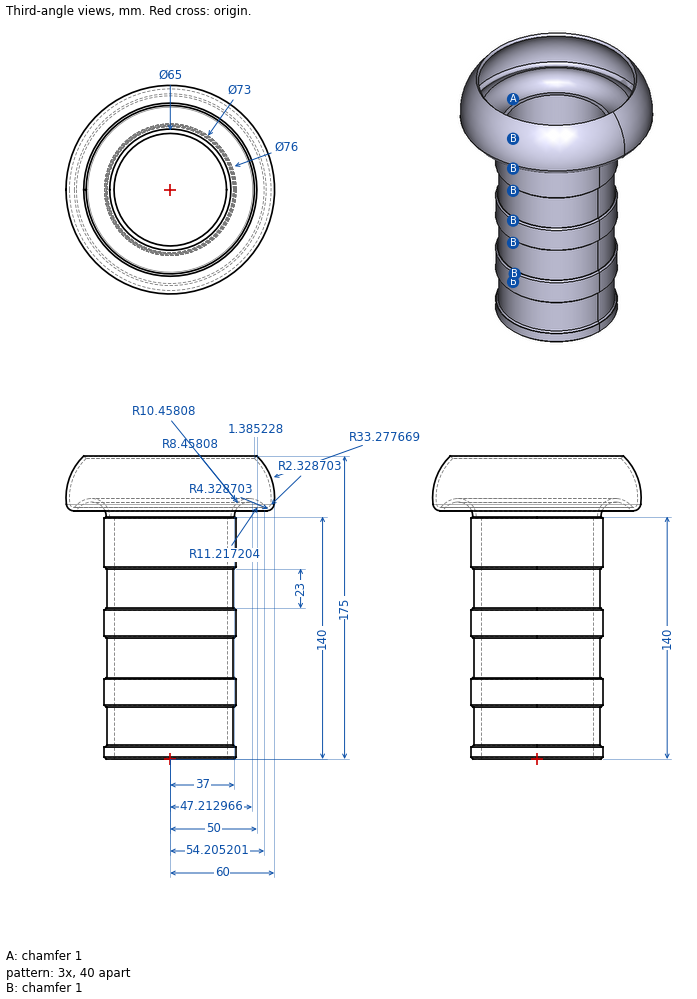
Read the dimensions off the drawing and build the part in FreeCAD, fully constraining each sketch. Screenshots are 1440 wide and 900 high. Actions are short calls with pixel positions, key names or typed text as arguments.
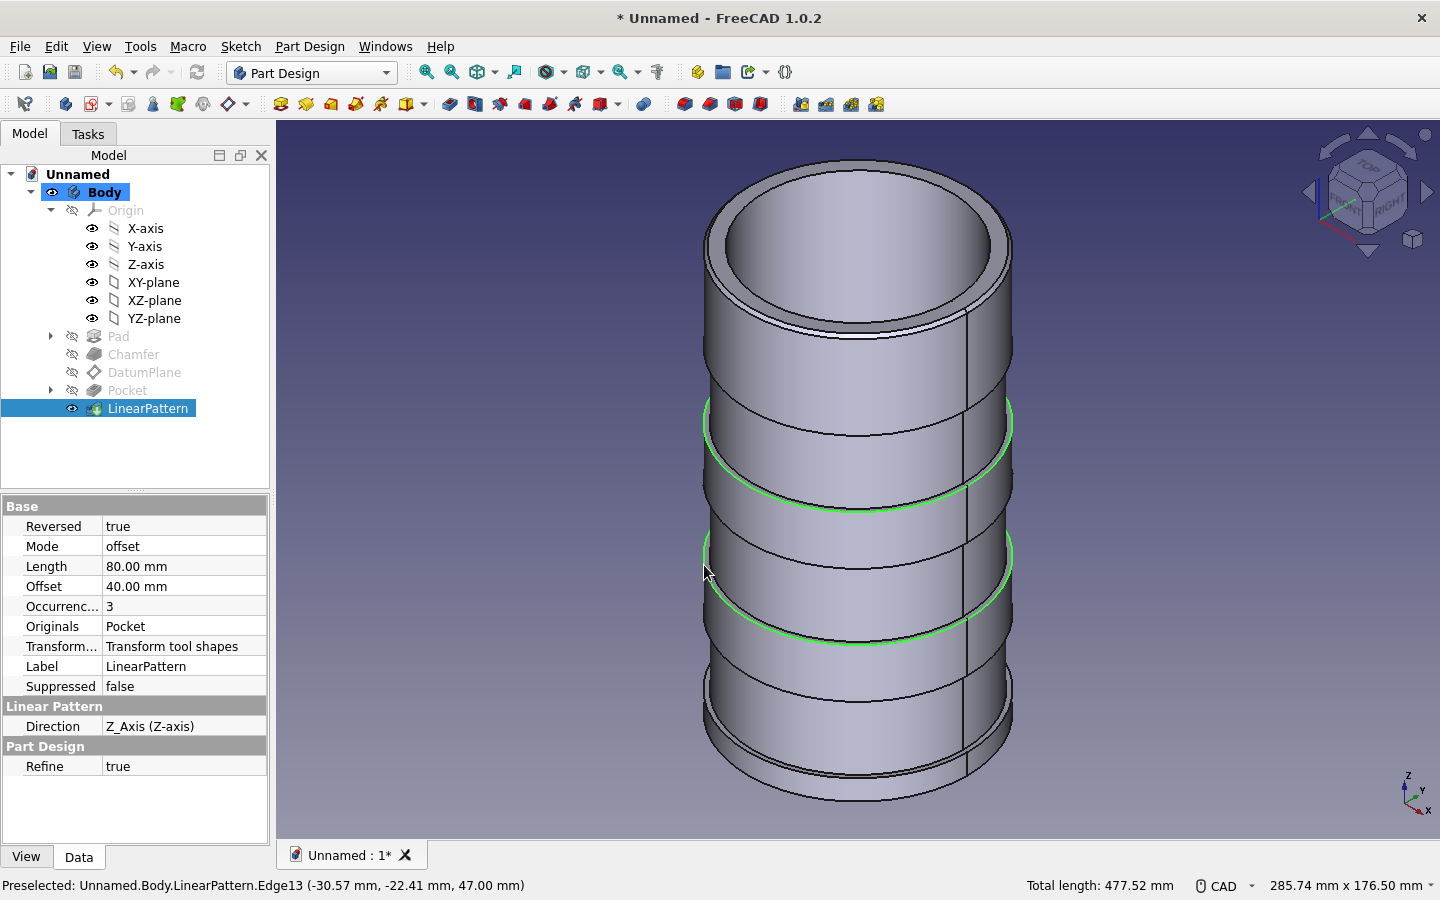
key(v)
key(f)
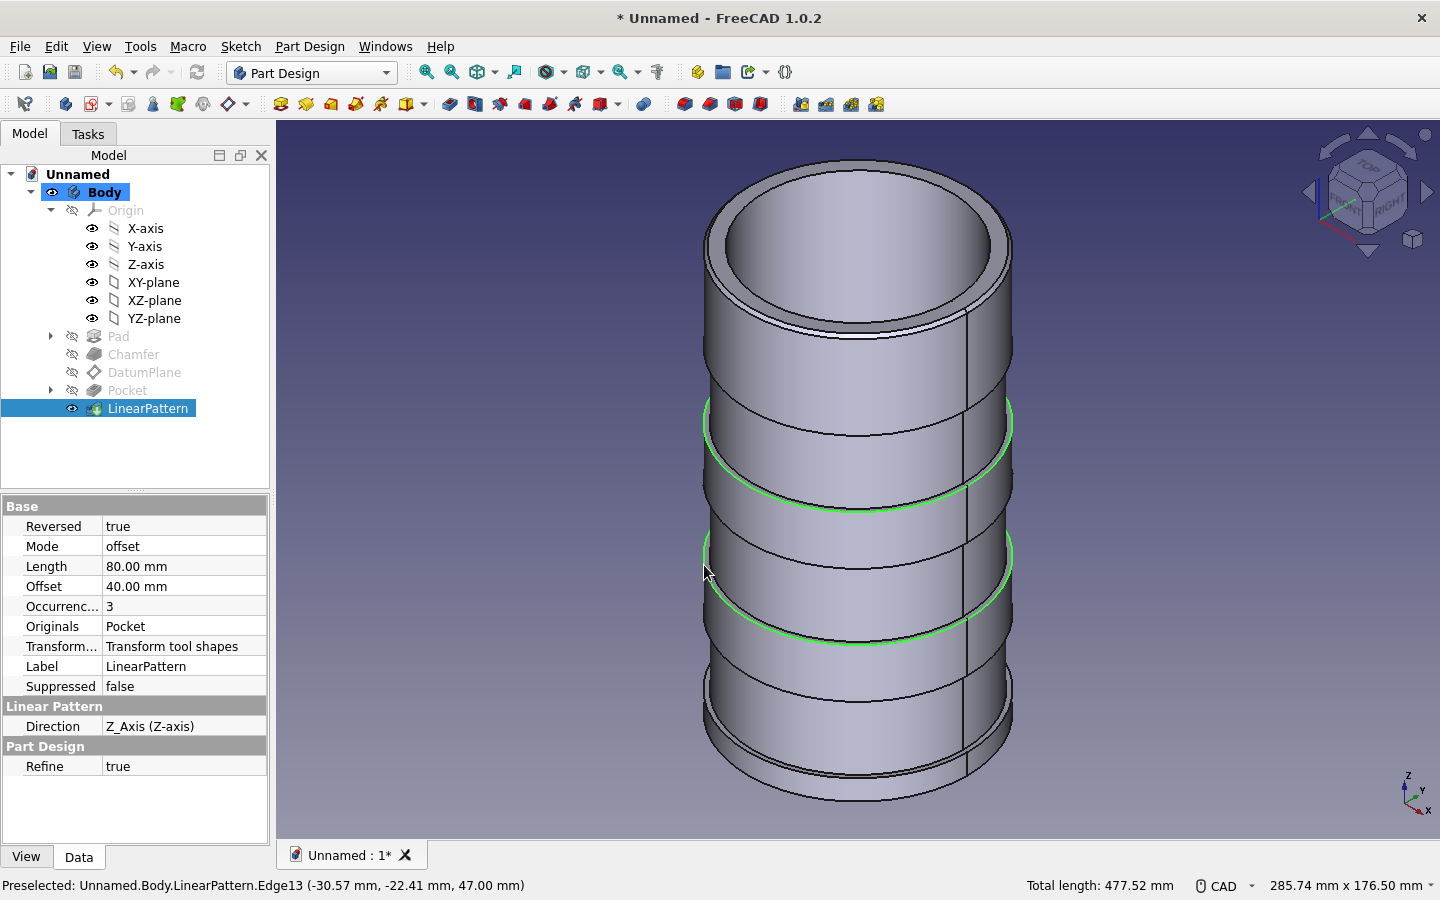
click(720, 386, ctrl)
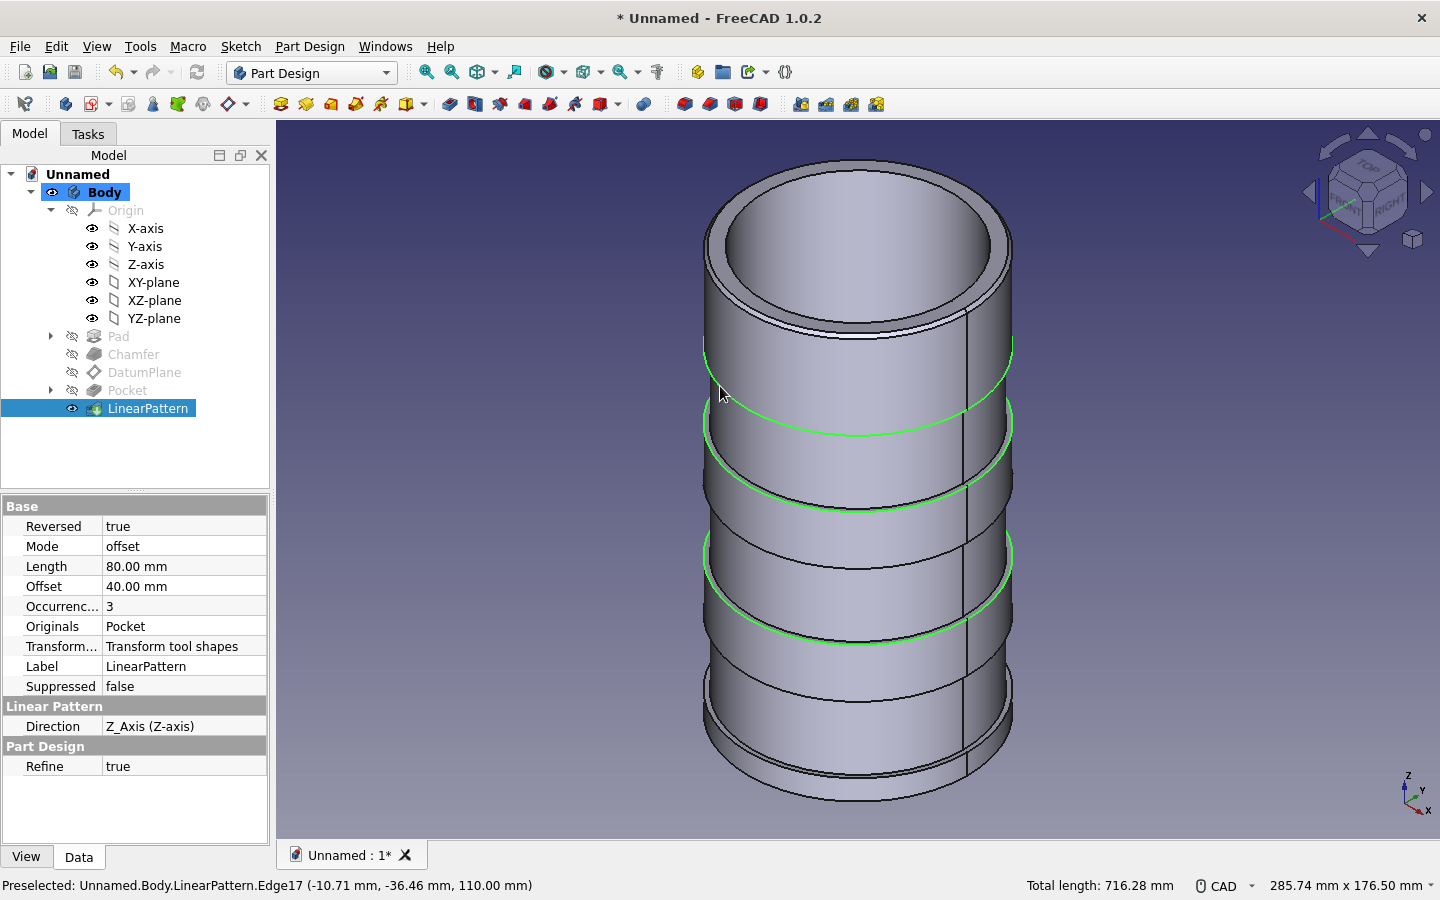
click(720, 752, ctrl)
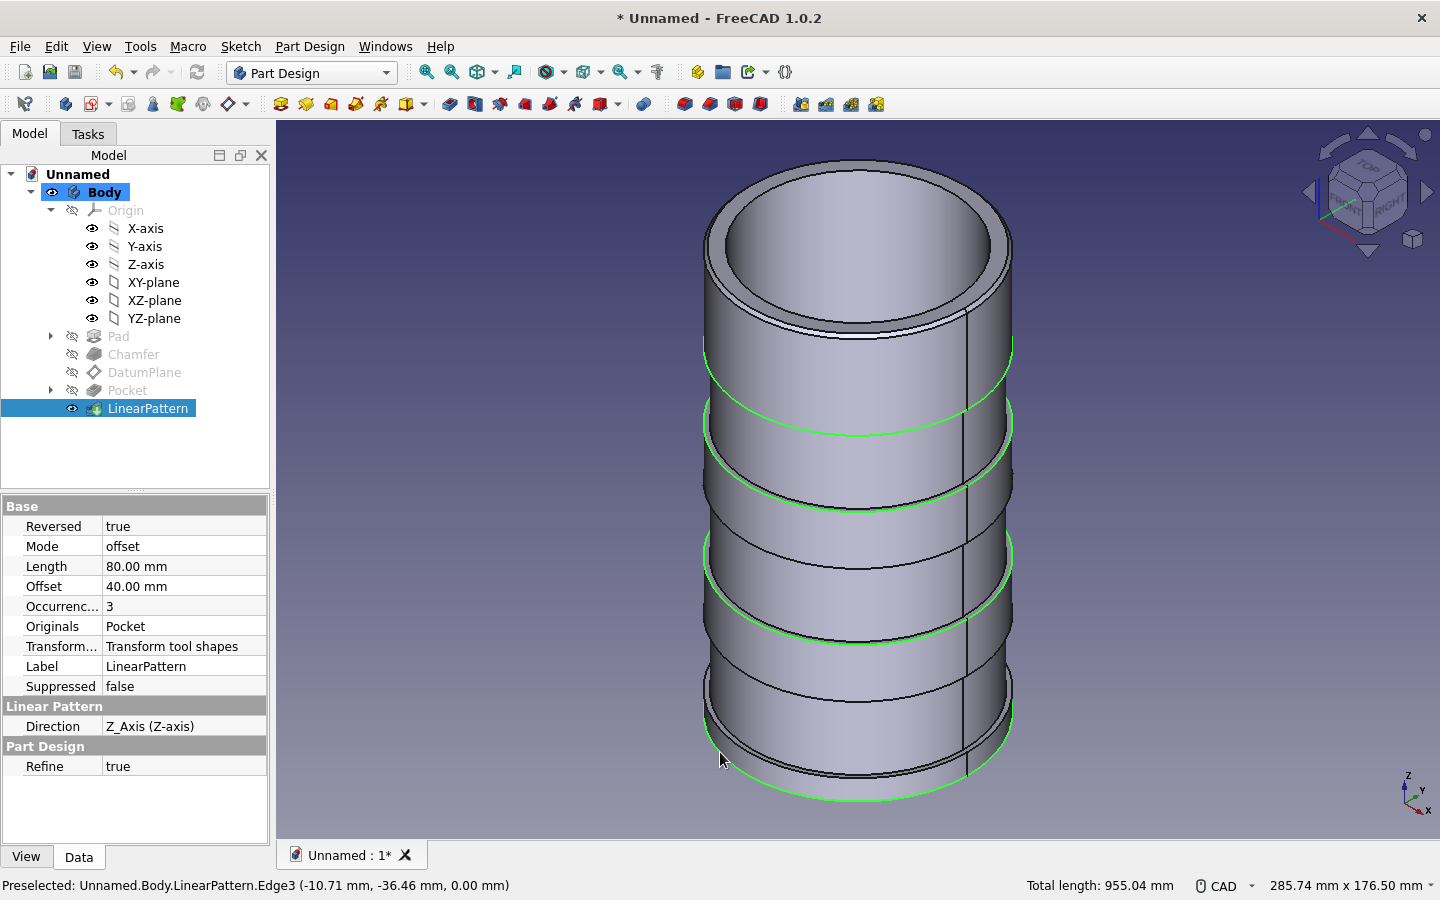
click(720, 519, ctrl)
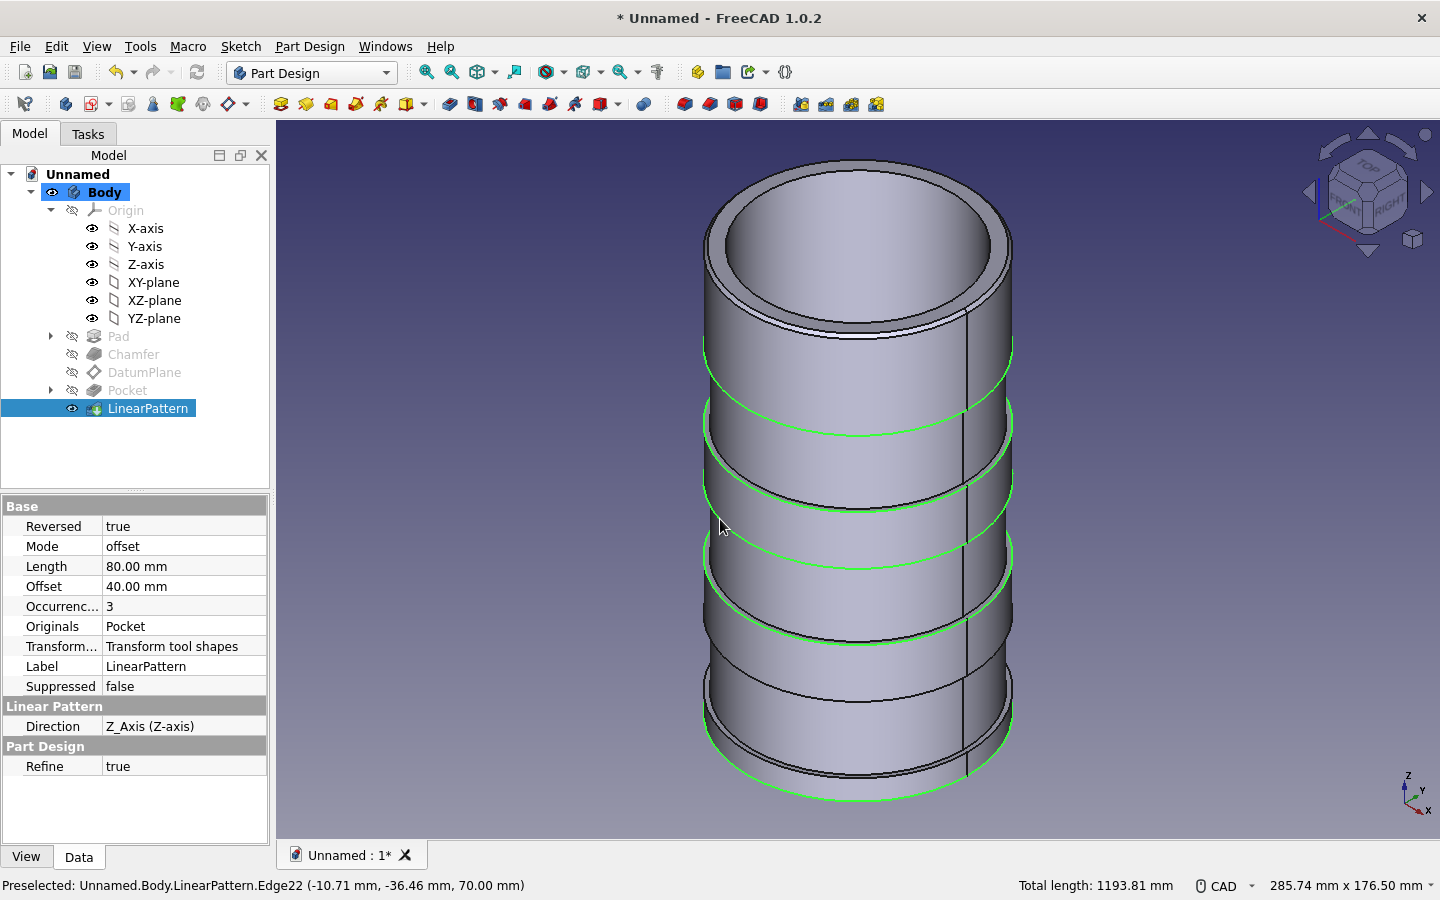
click(720, 652, ctrl)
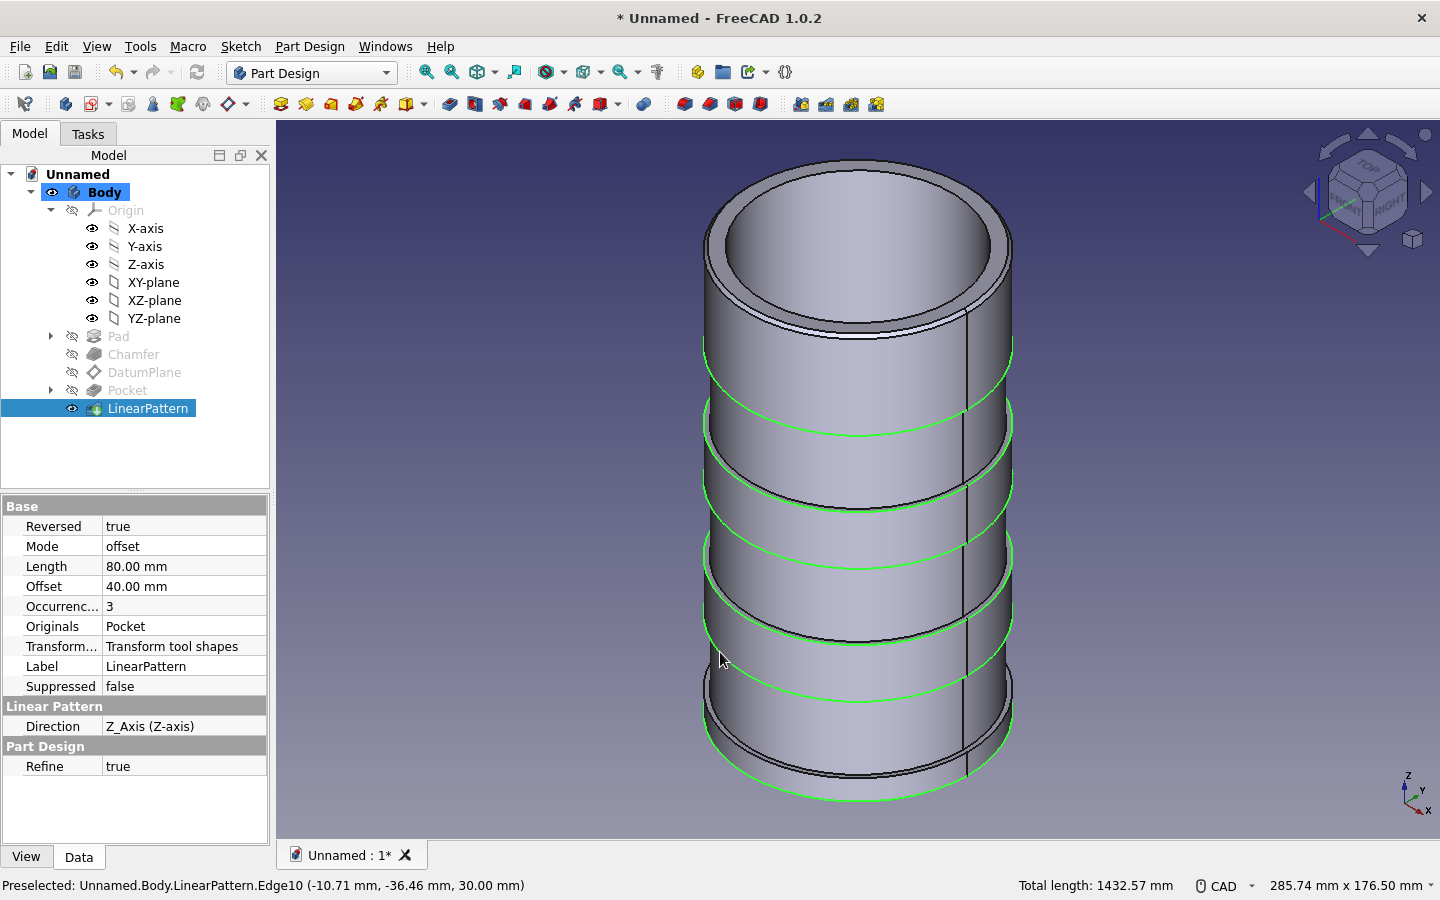
key(2)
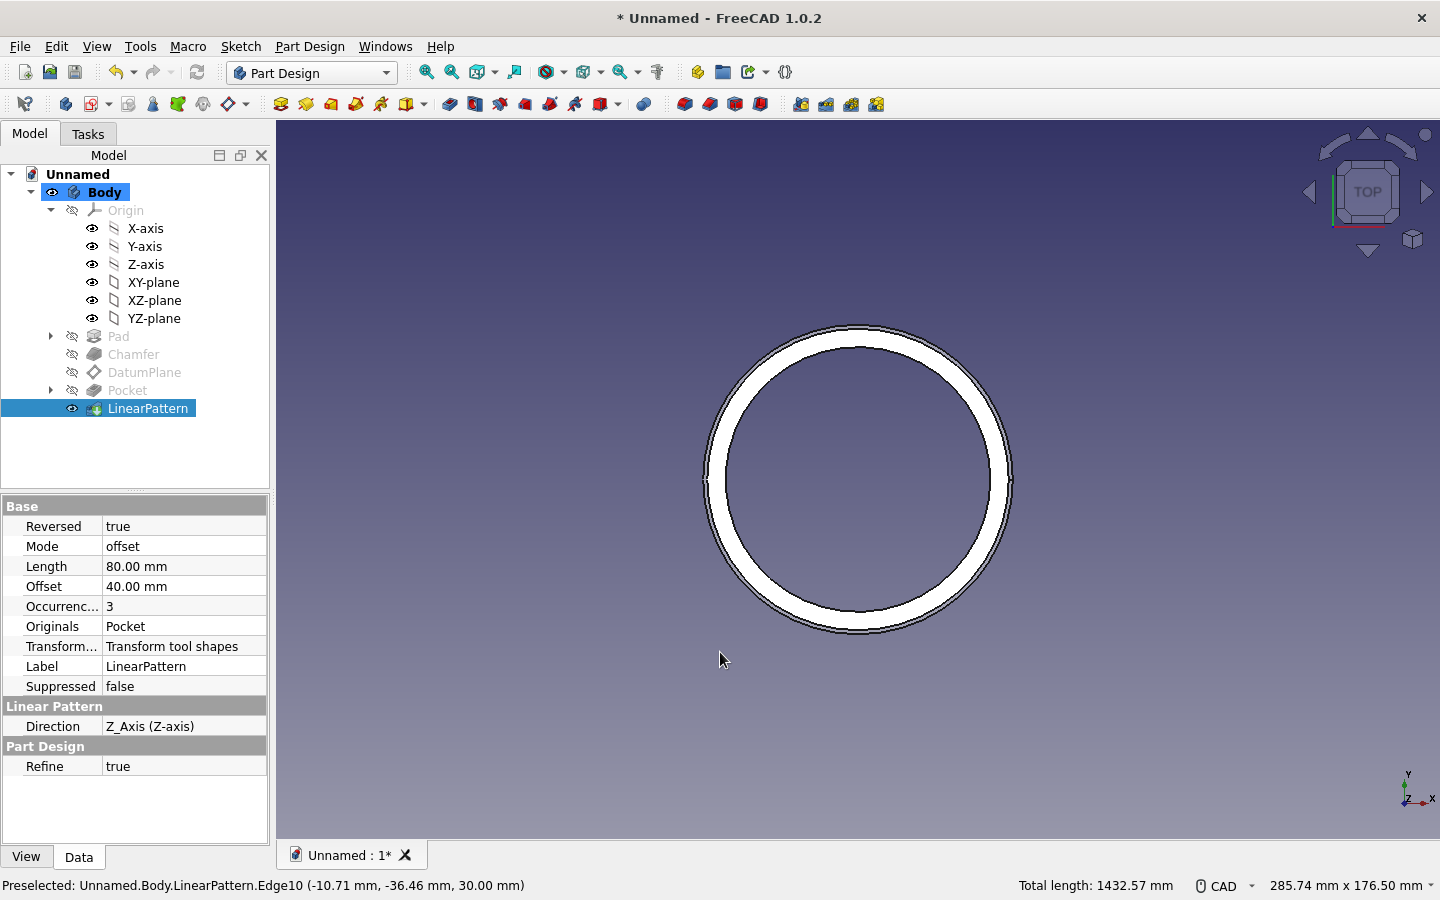
key(v)
key(f)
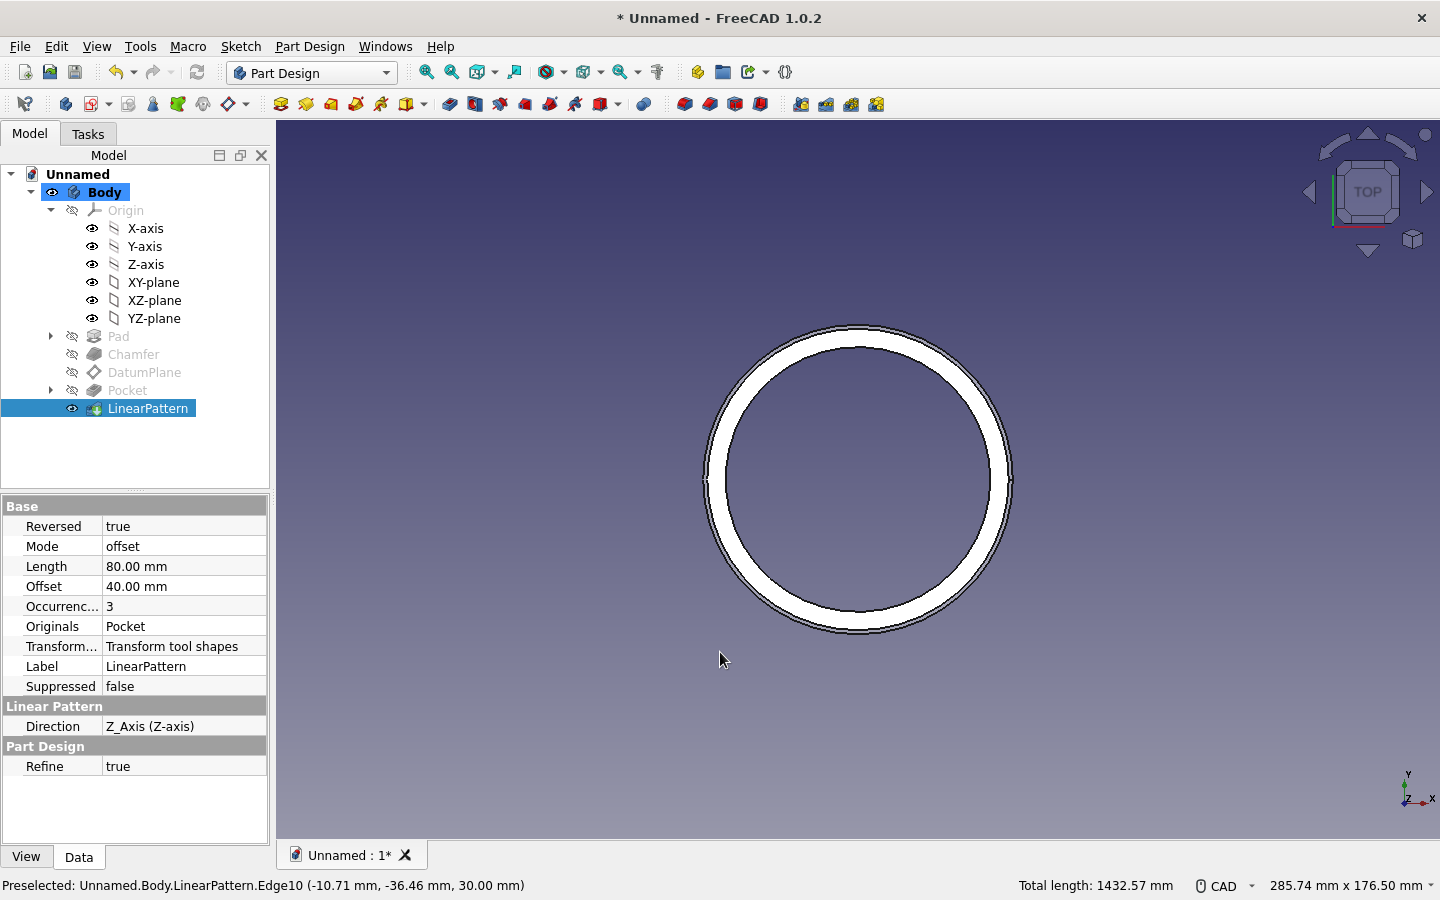
key(1)